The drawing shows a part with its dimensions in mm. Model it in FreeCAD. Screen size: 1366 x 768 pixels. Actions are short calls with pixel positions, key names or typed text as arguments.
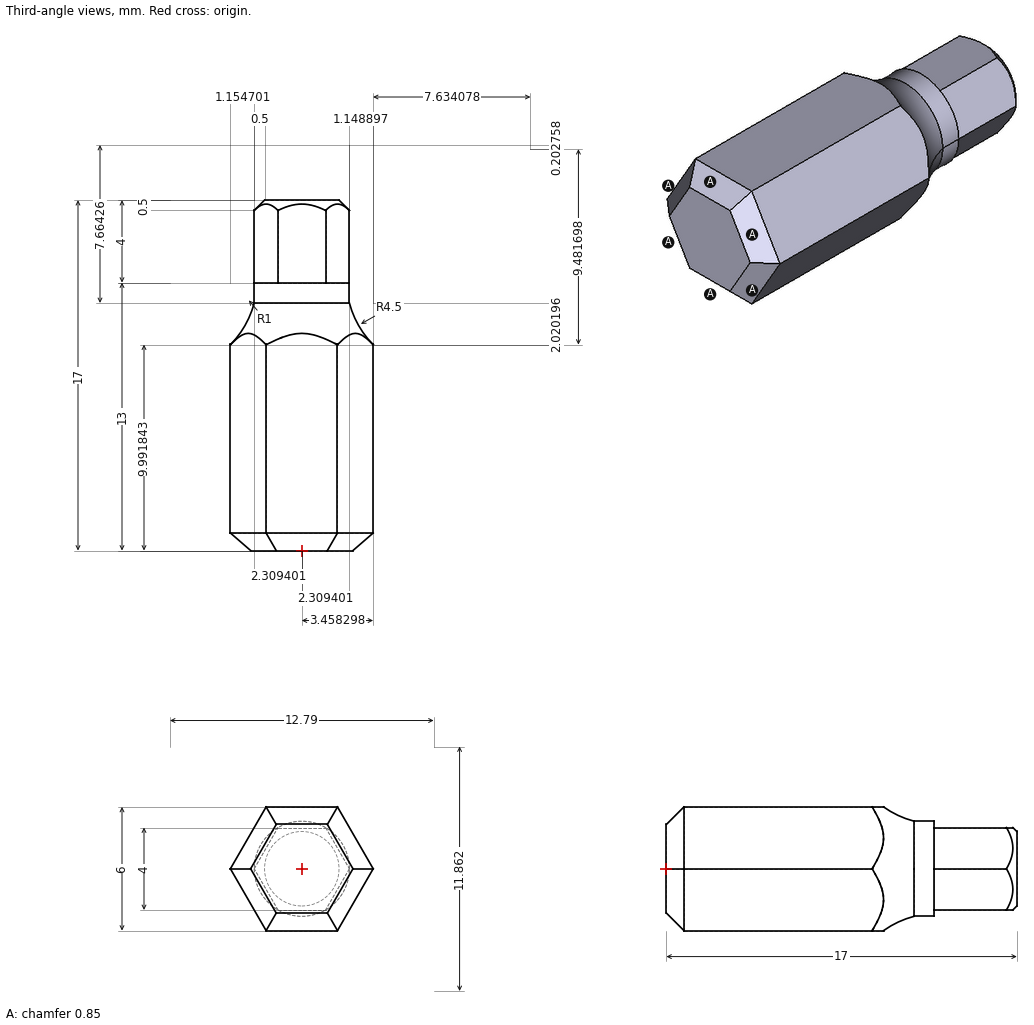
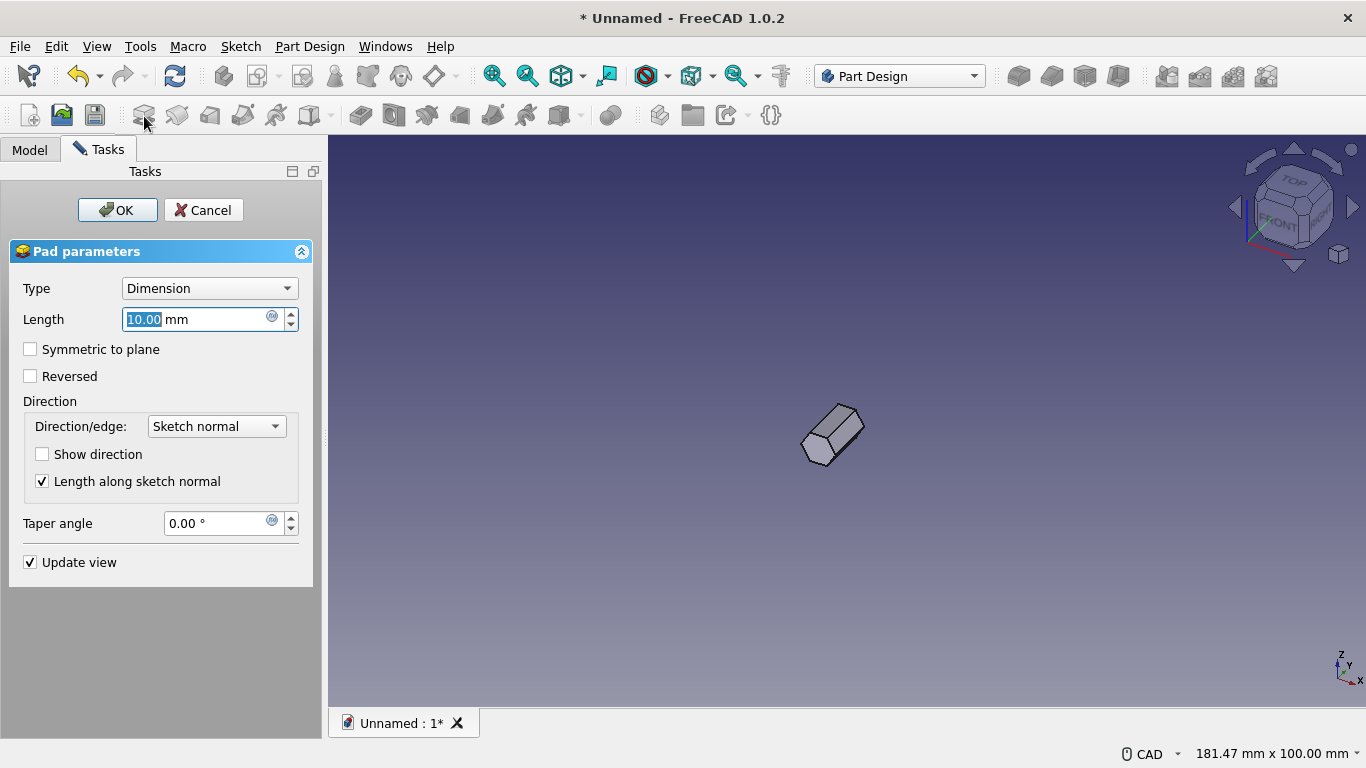
text(17)
key(Tab)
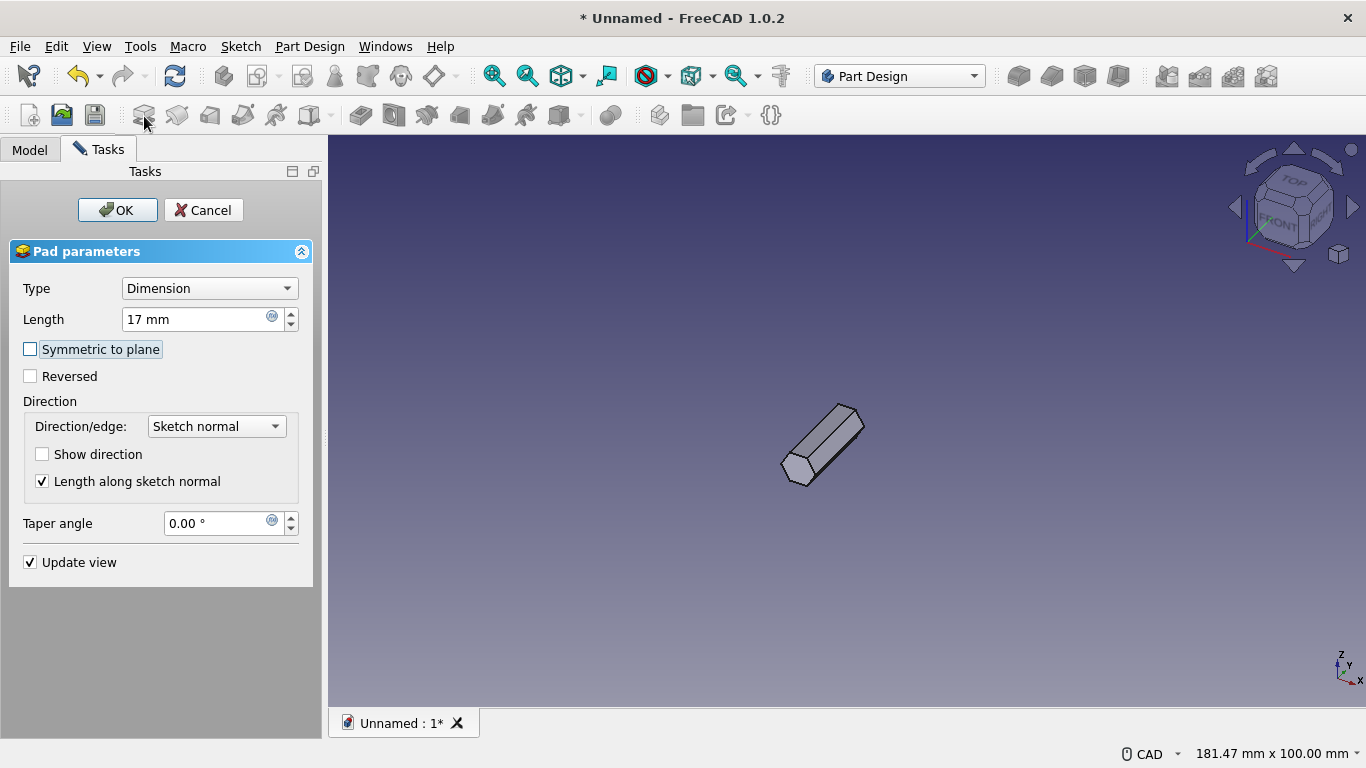
click(31, 376)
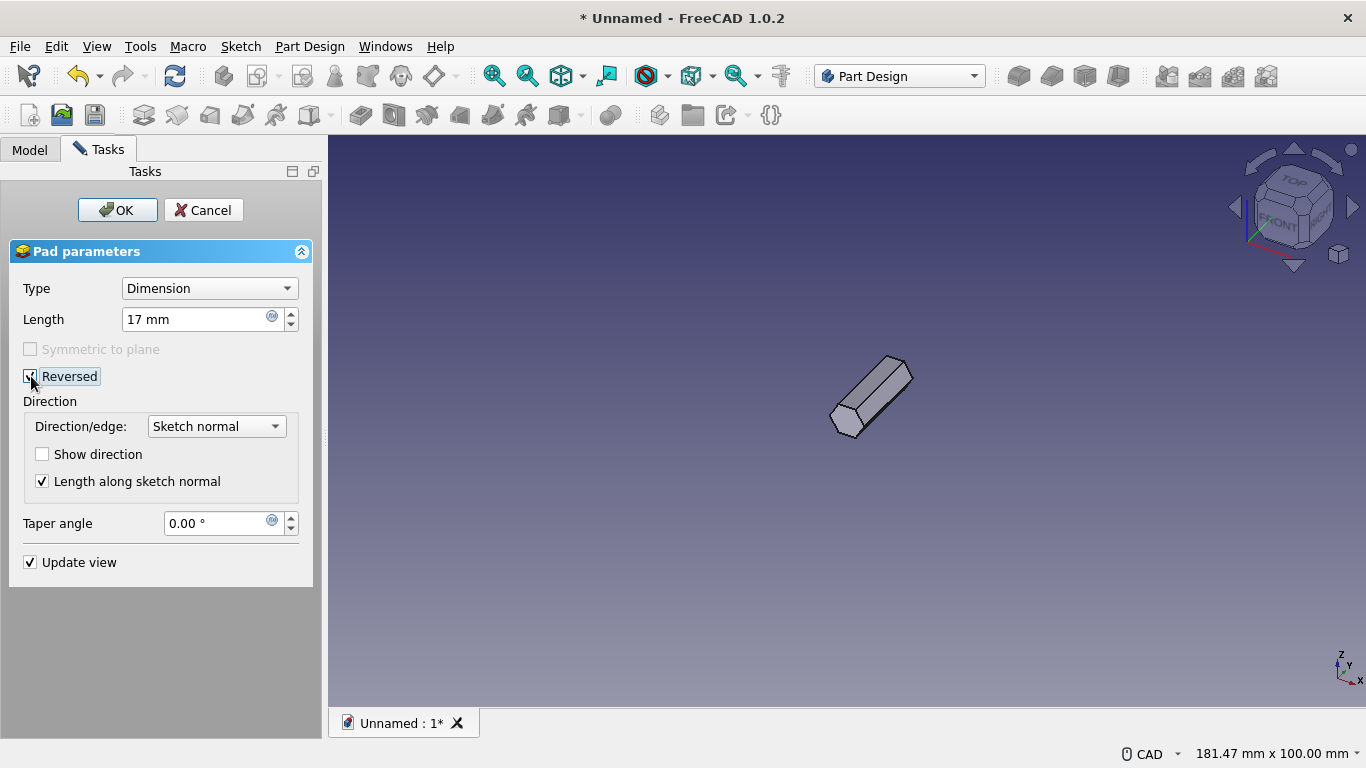
click(118, 210)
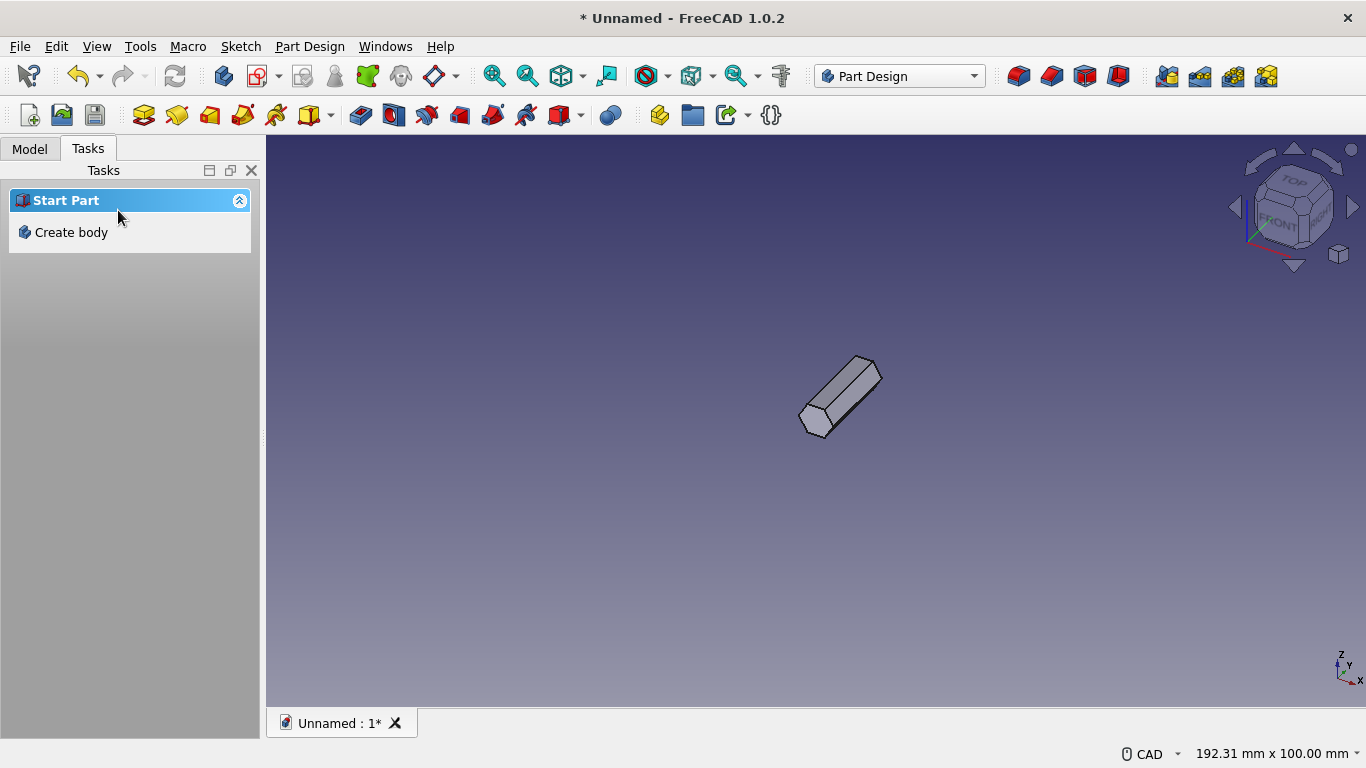
click(495, 76)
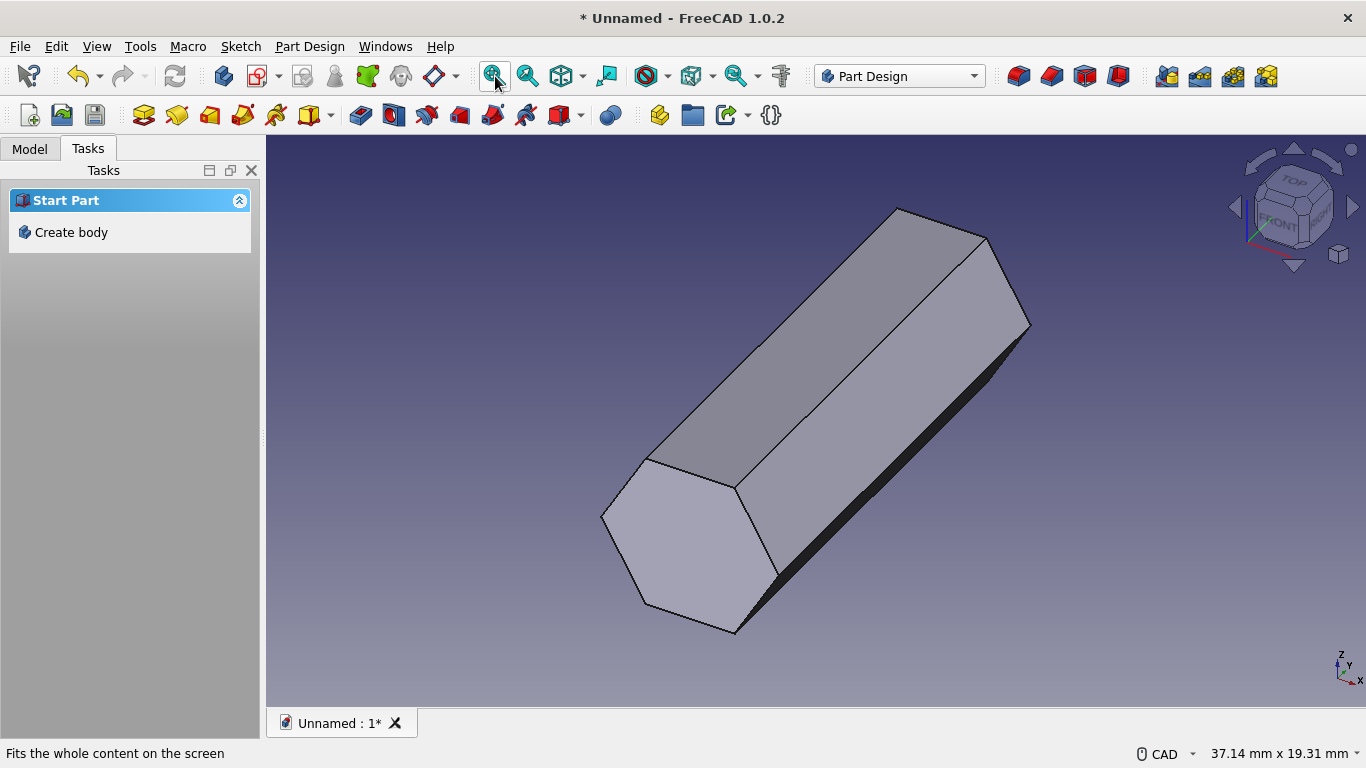
click(690, 545)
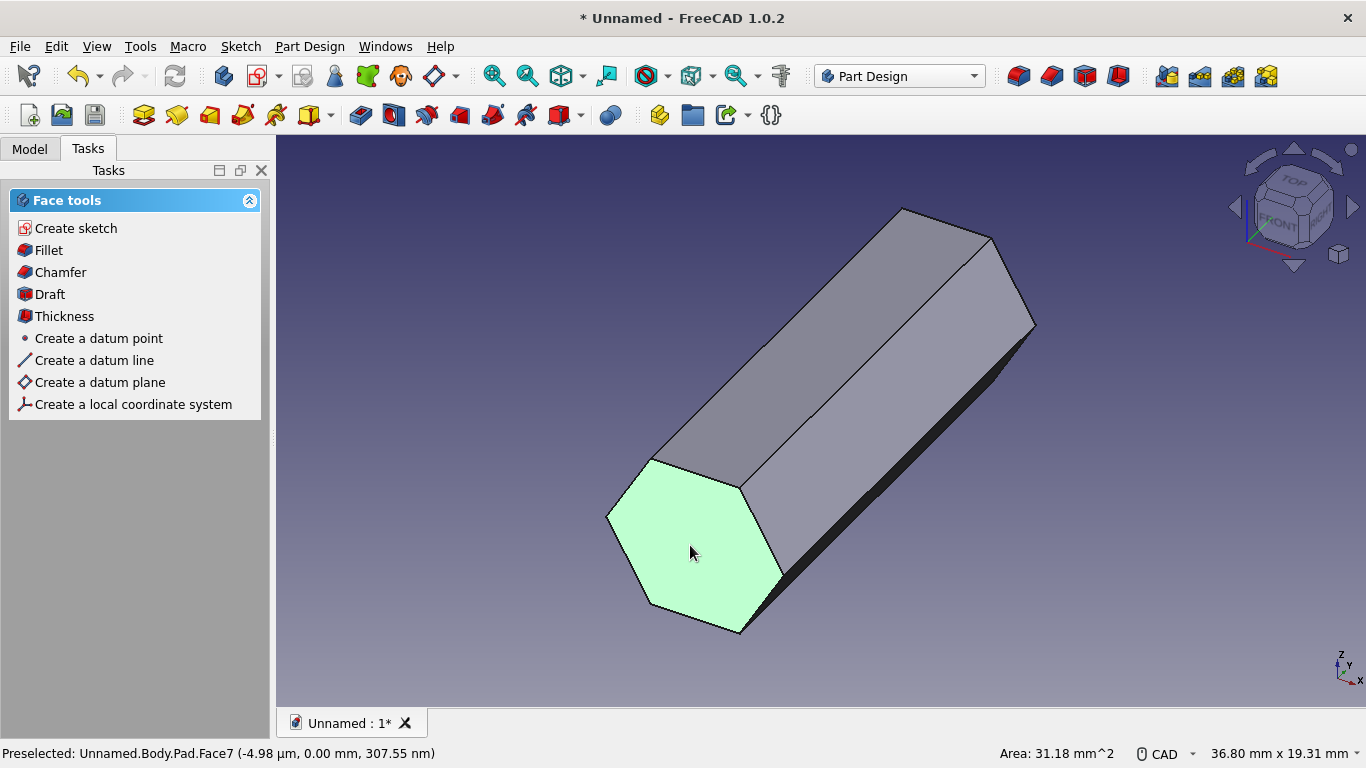
click(1052, 76)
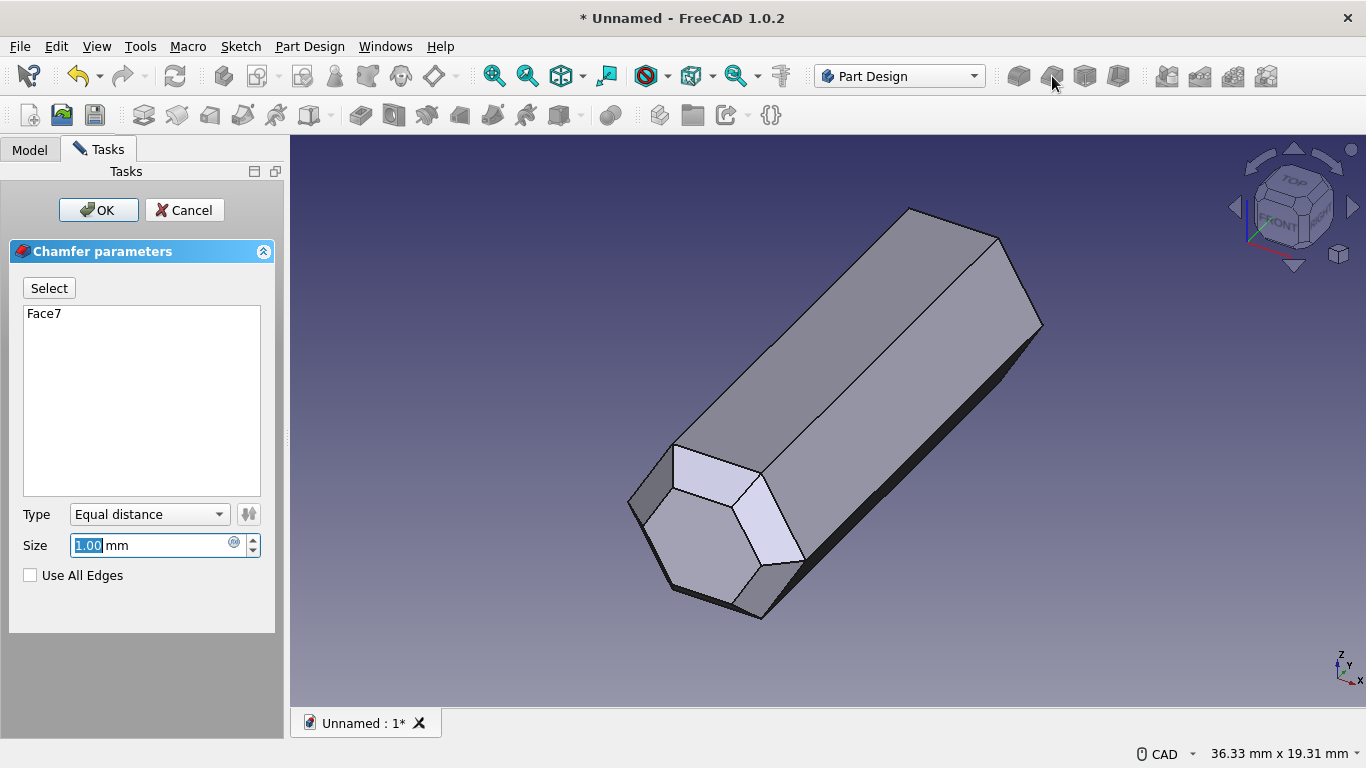
text(0.85)
key(Tab)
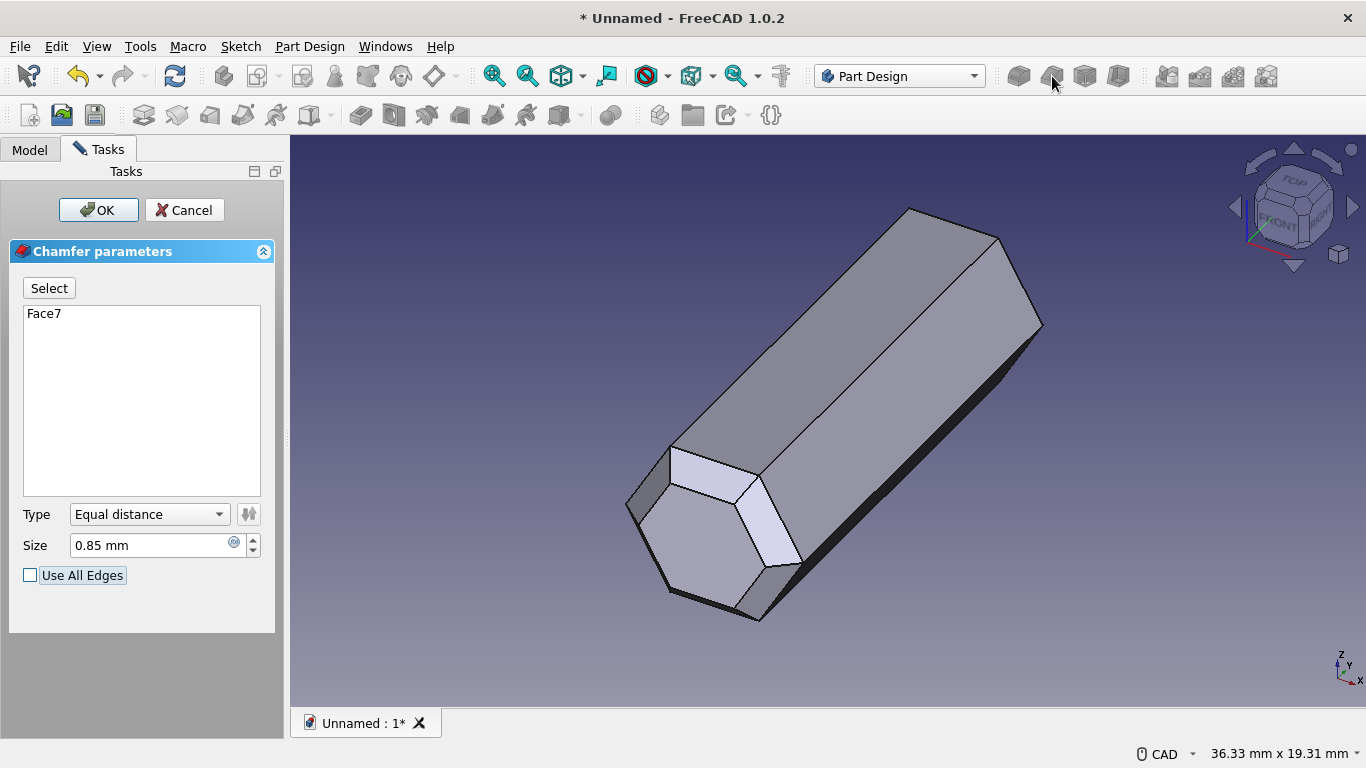
click(99, 210)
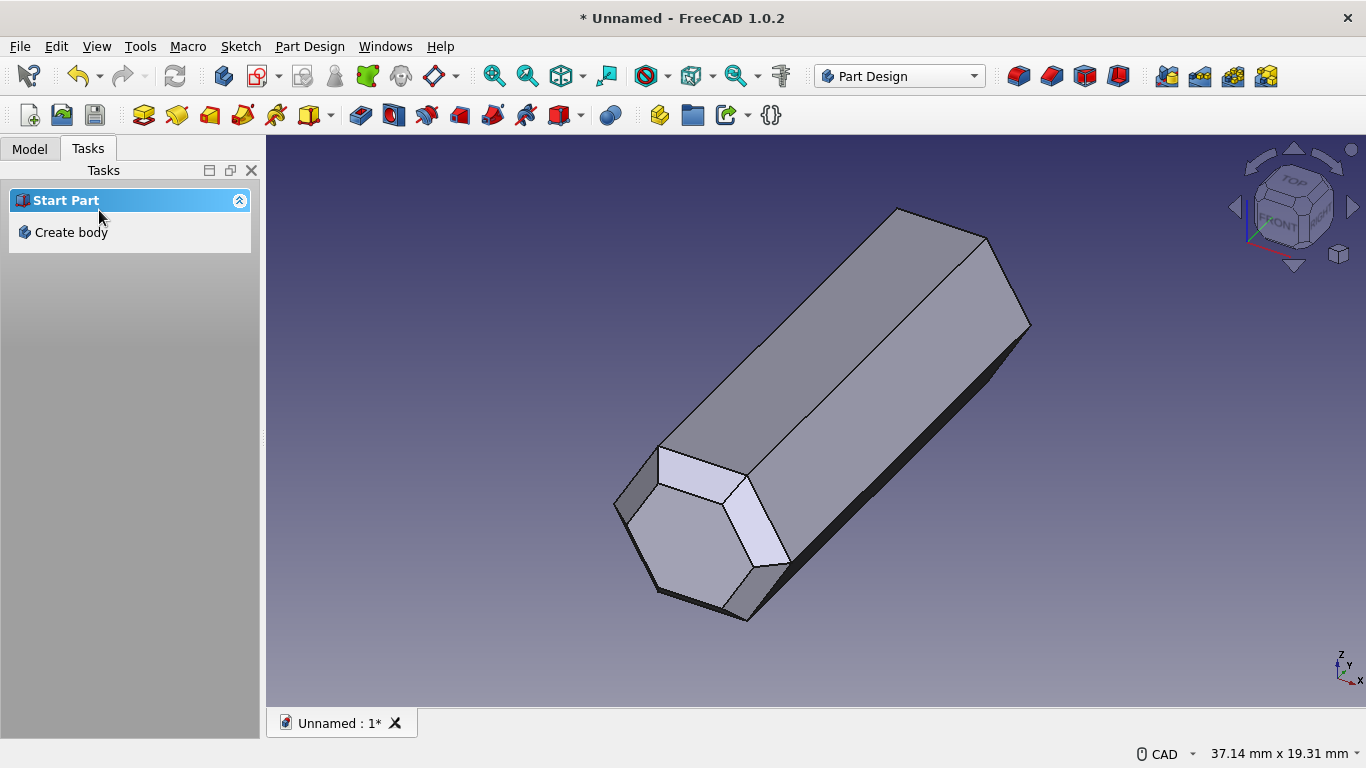
key(4)